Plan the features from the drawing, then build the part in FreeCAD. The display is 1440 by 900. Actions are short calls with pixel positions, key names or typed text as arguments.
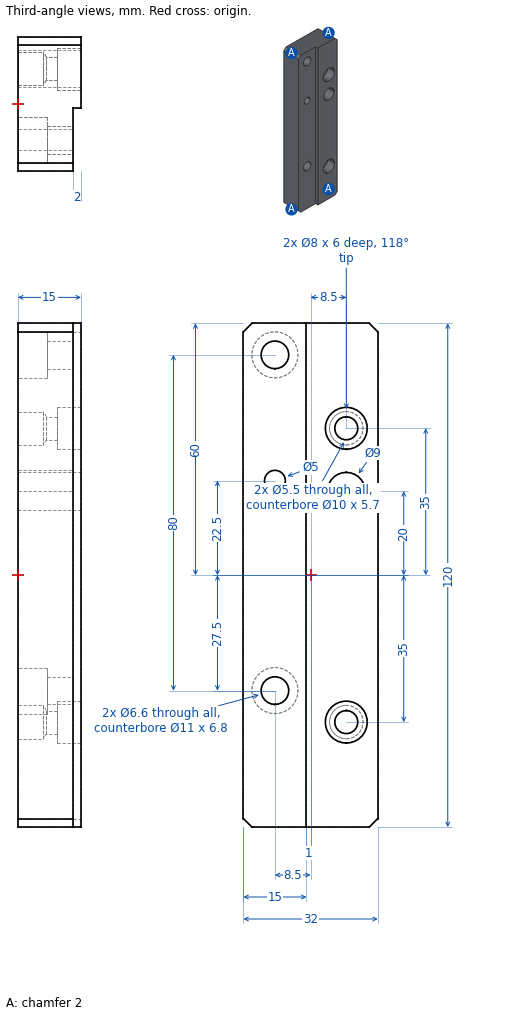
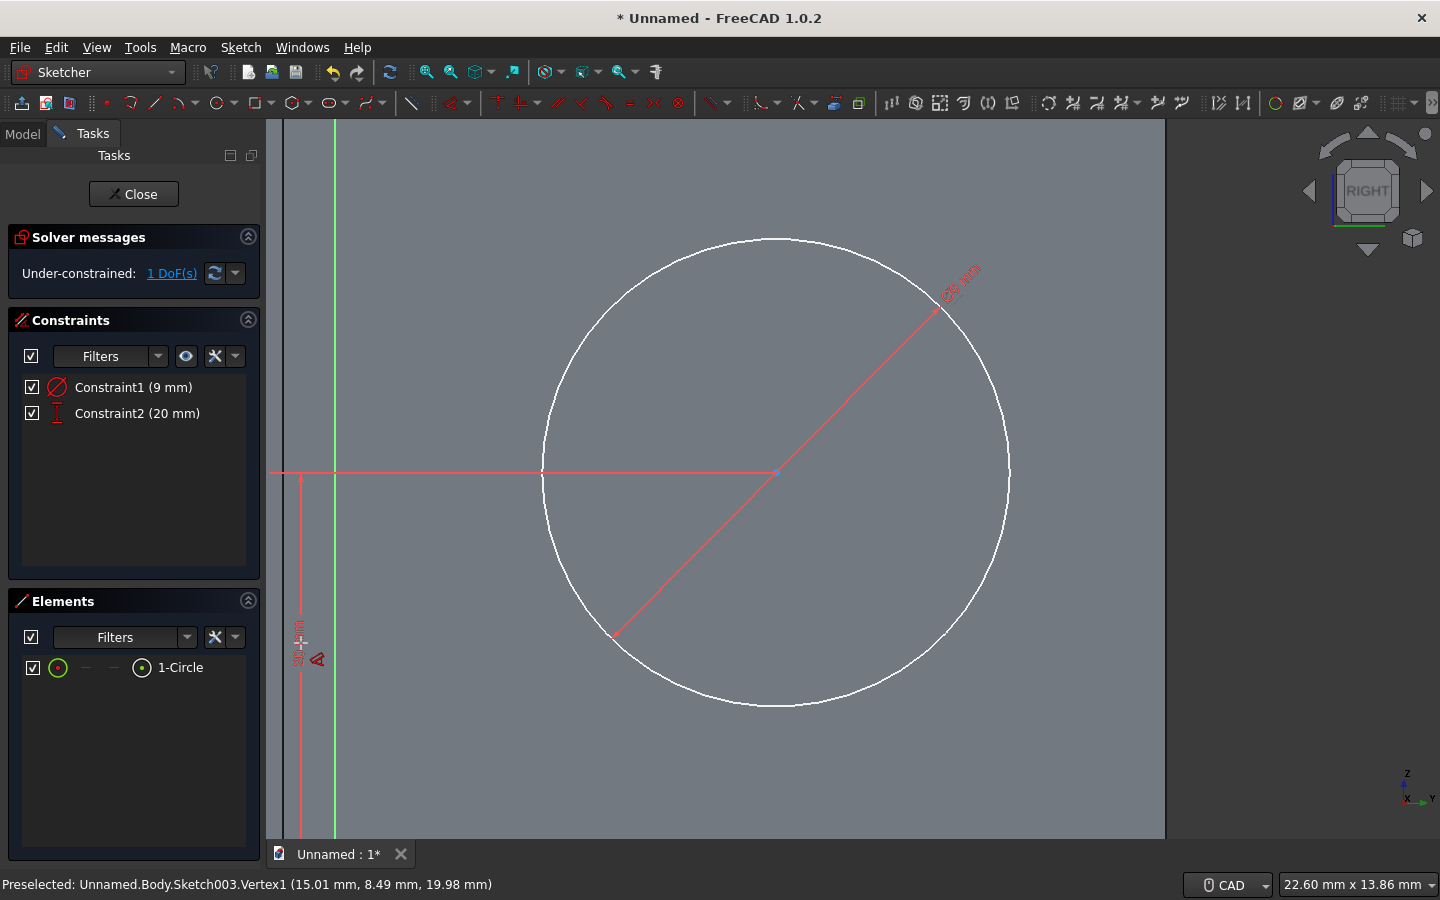
click(776, 473)
click(454, 439)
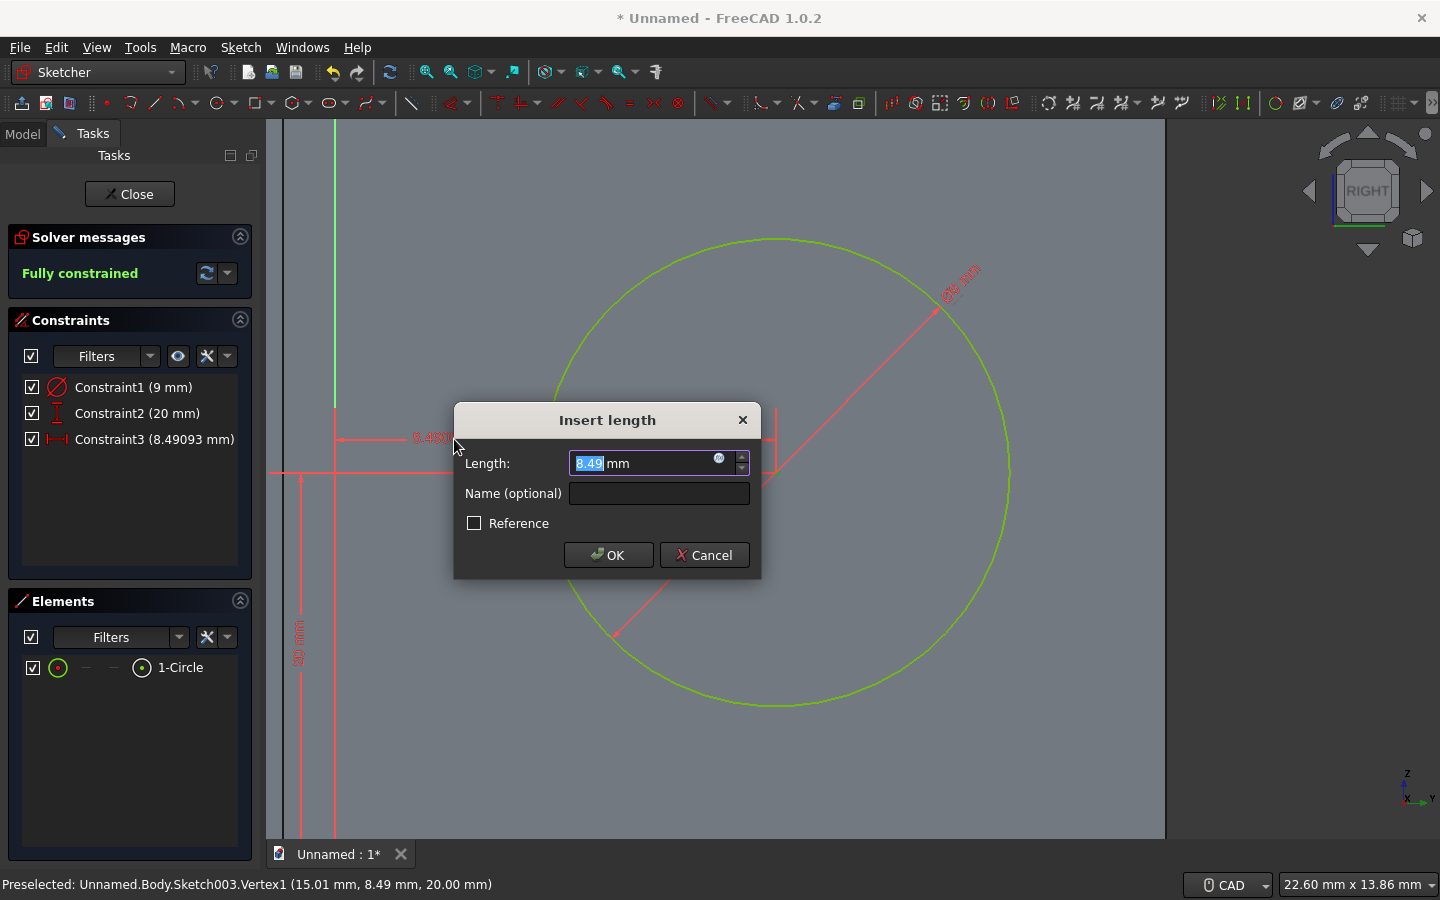
text(8.5)
key(Return)
key(Escape)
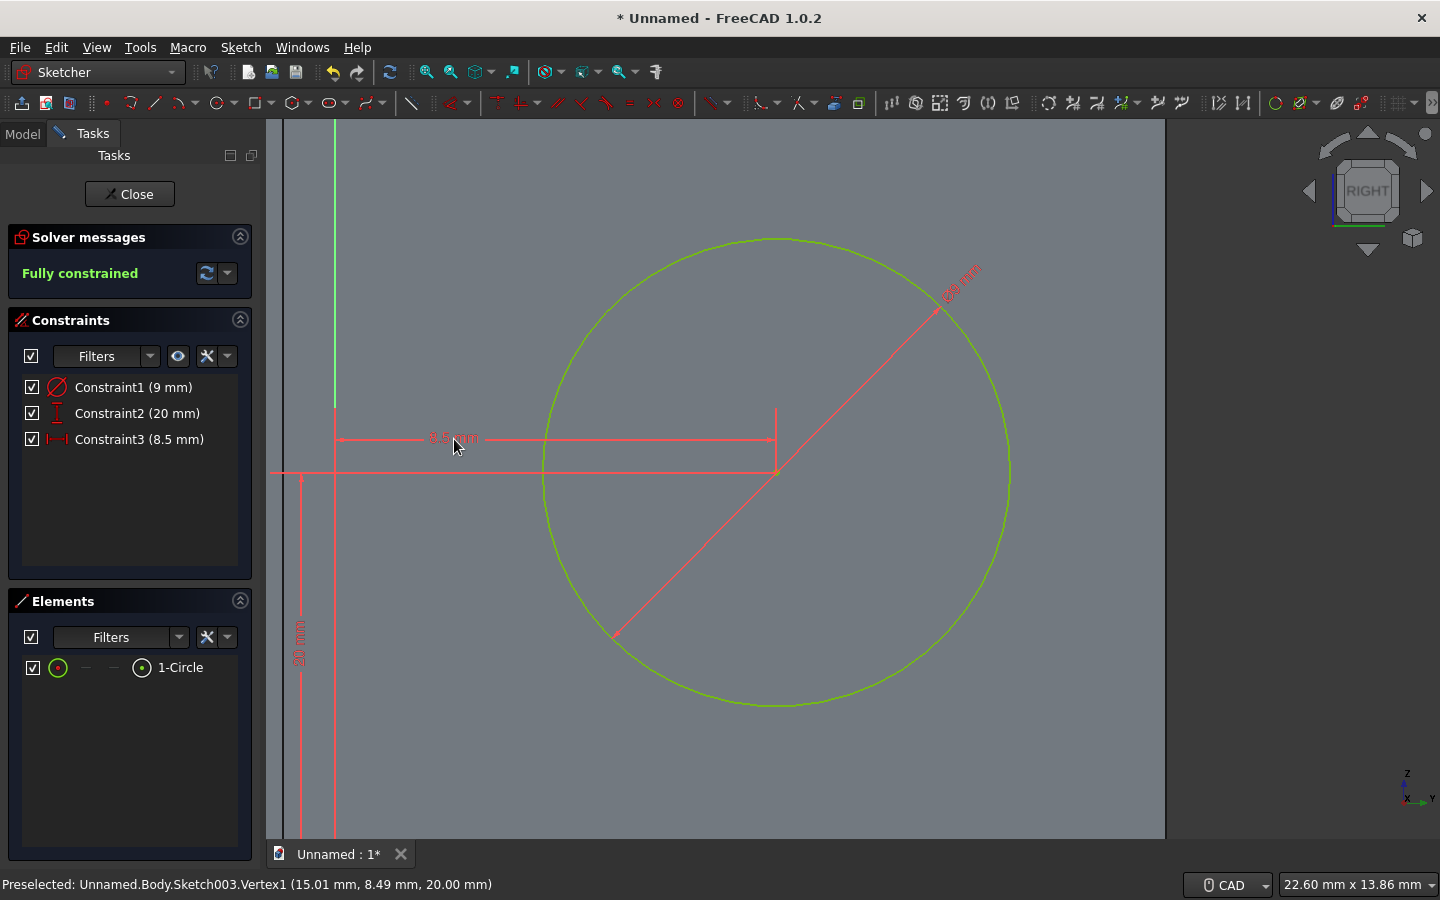
click(130, 194)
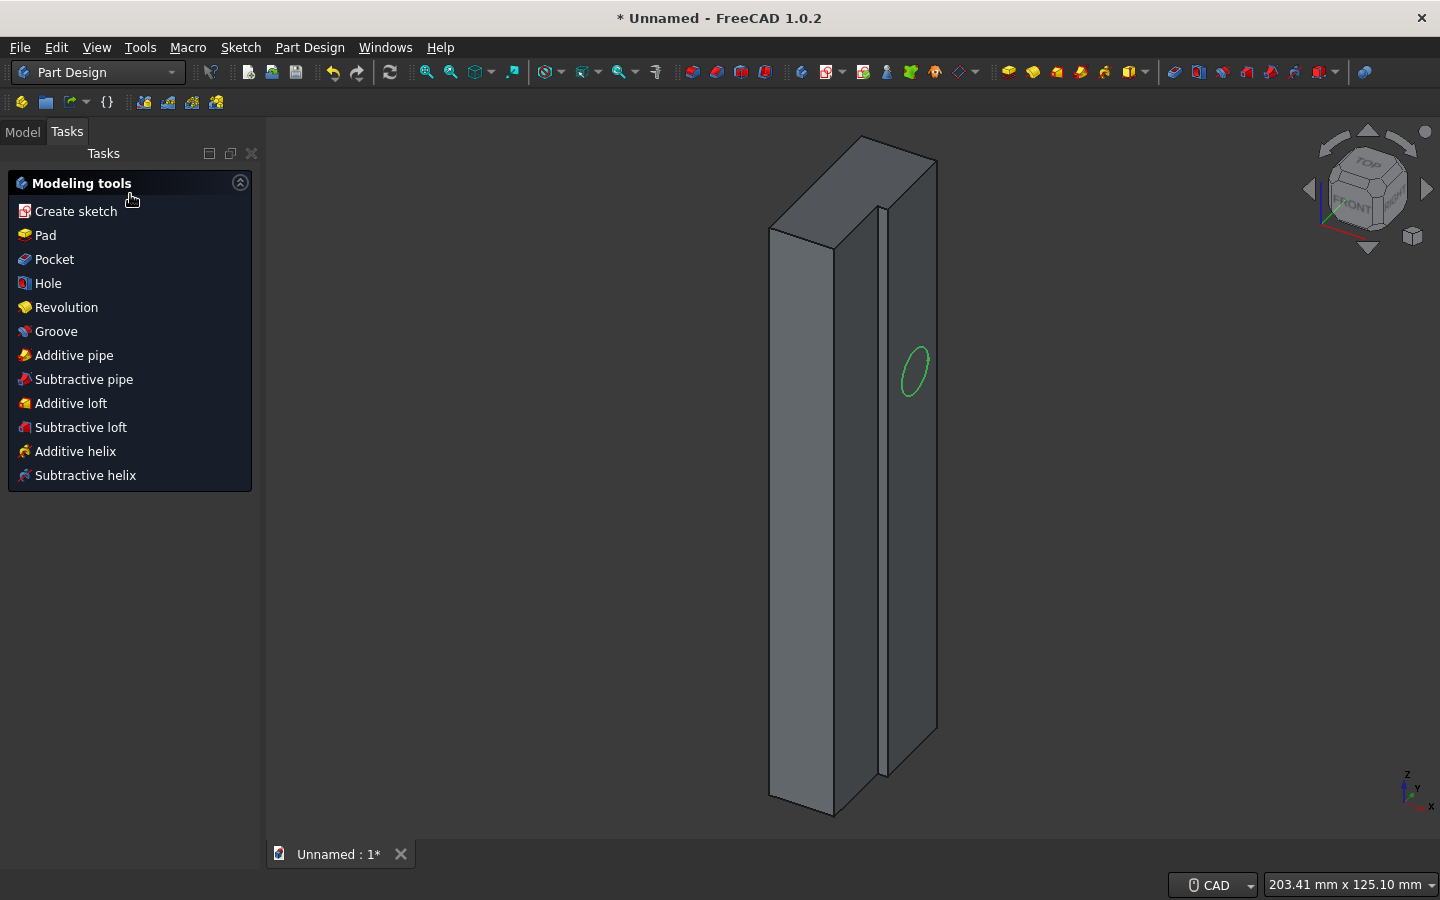
click(1176, 72)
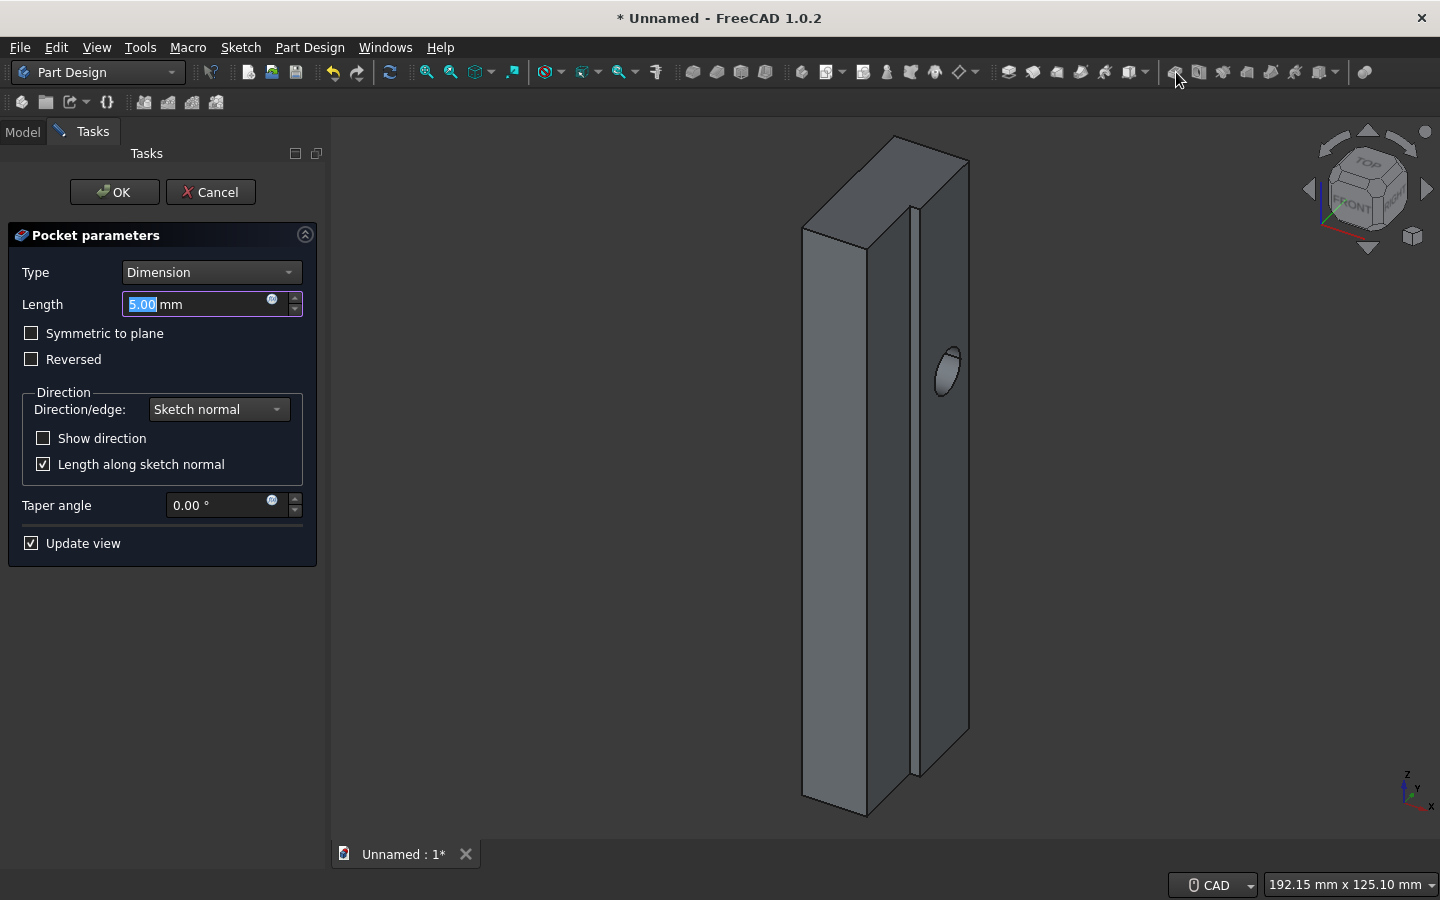
click(212, 272)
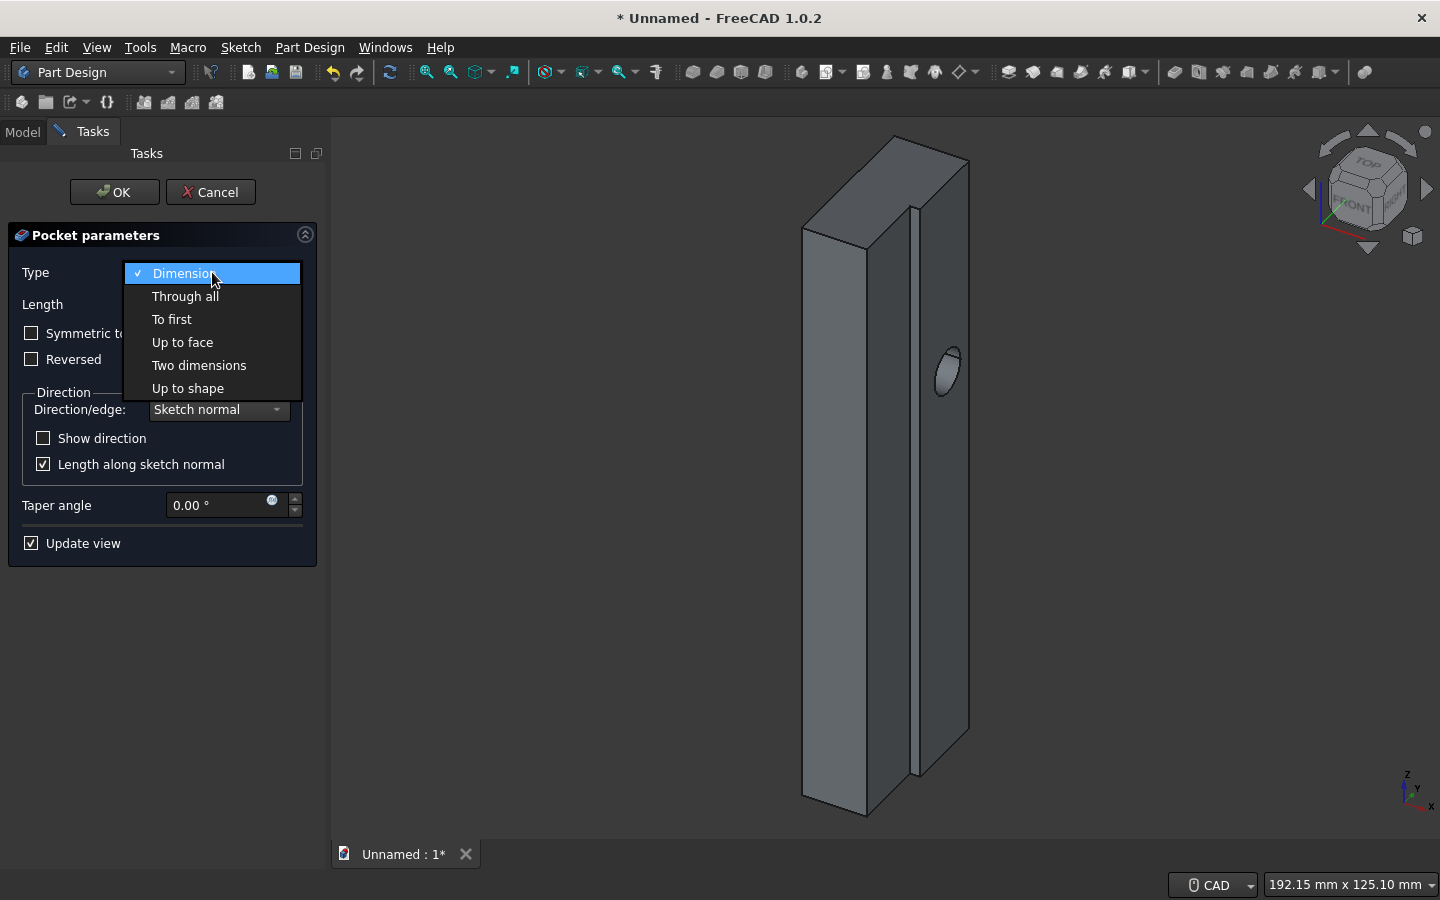
click(212, 296)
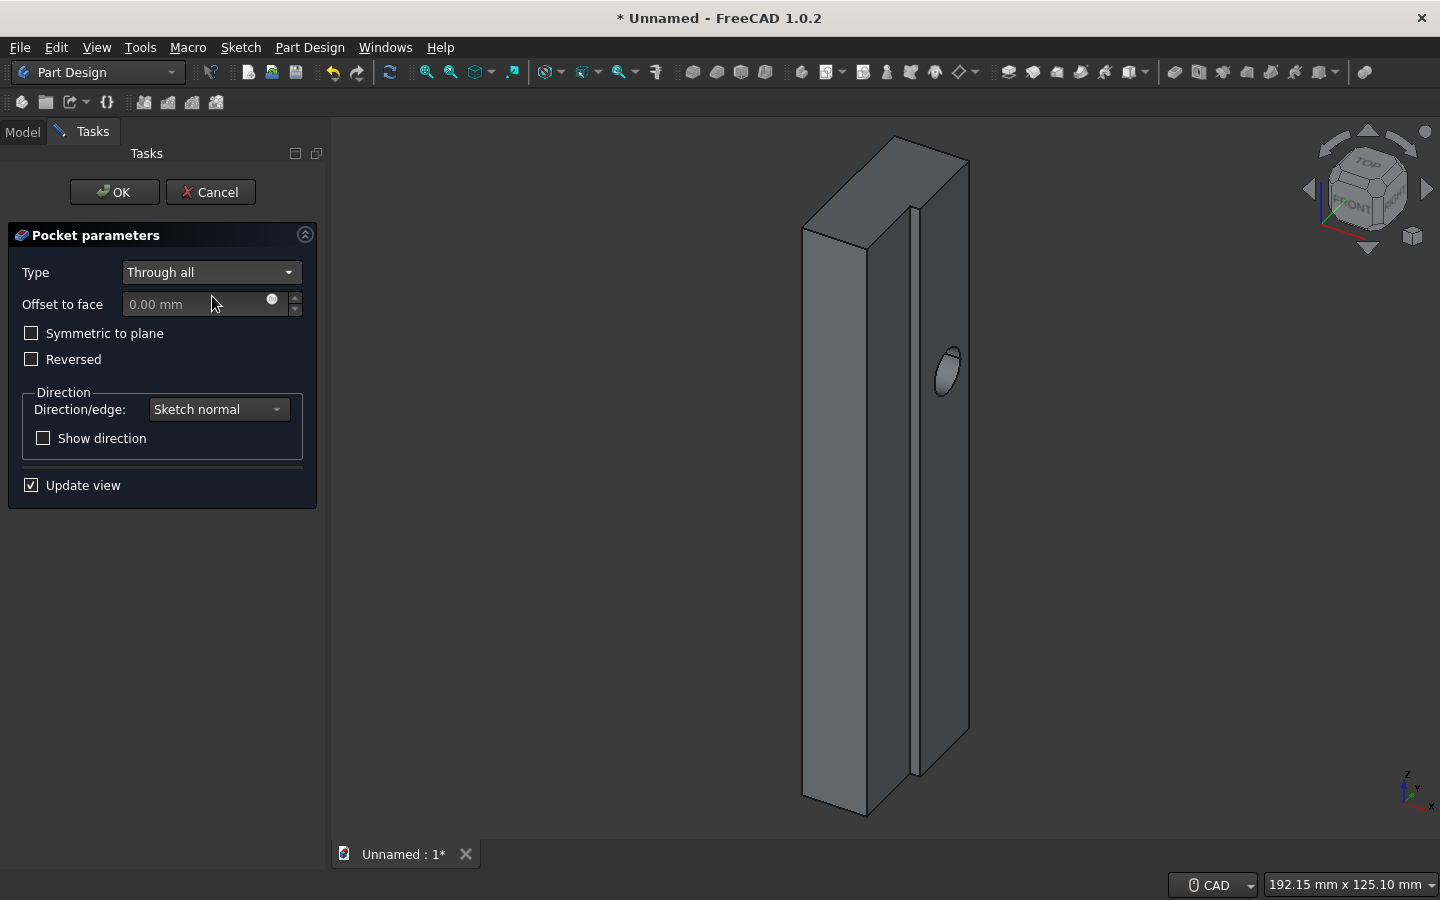
click(115, 192)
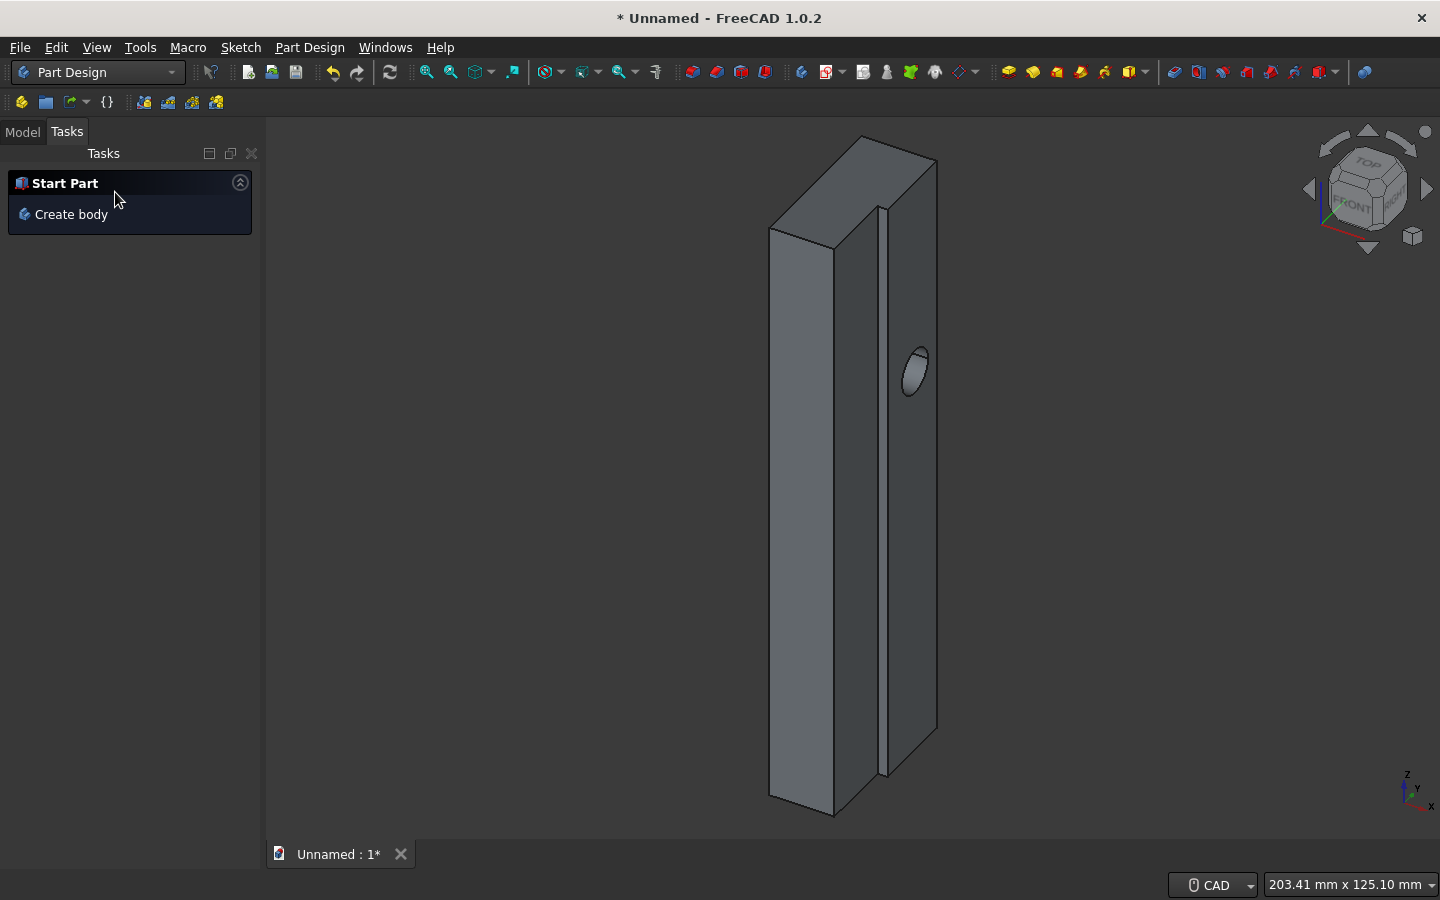
click(802, 238)